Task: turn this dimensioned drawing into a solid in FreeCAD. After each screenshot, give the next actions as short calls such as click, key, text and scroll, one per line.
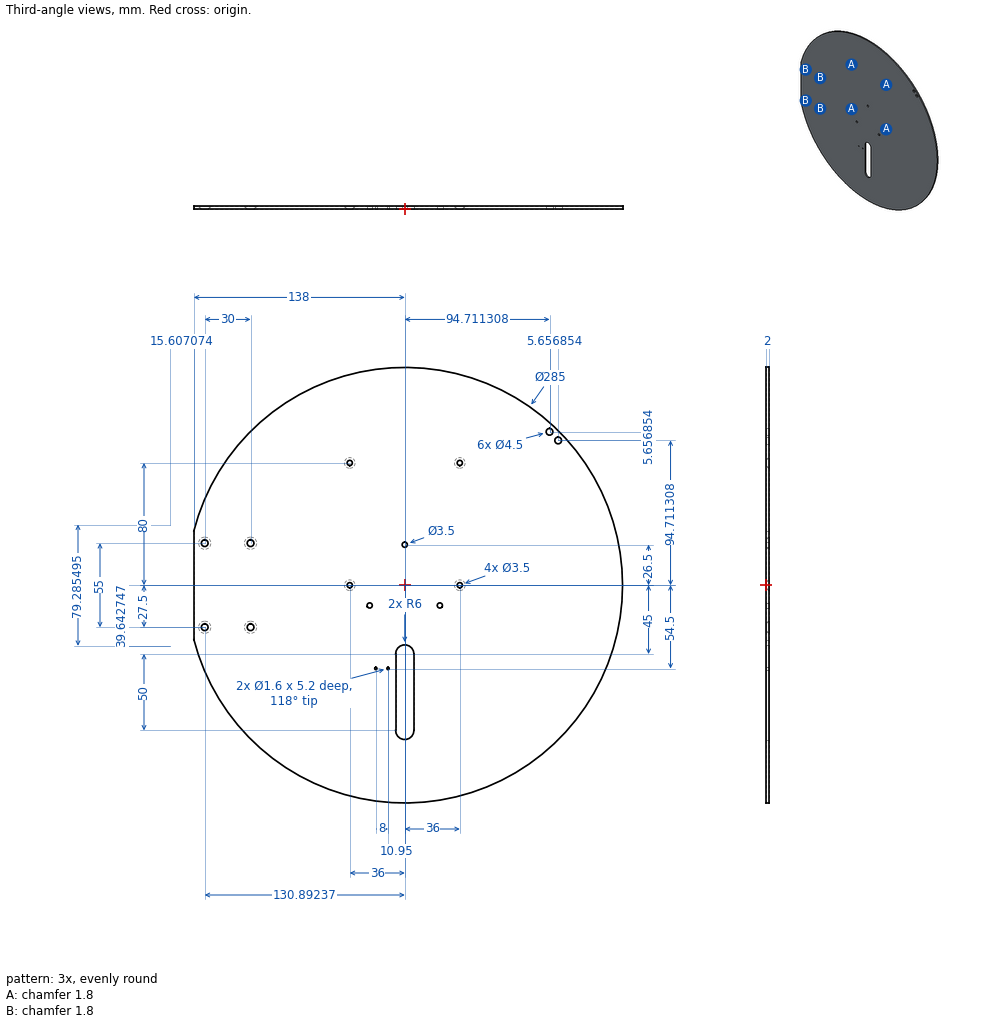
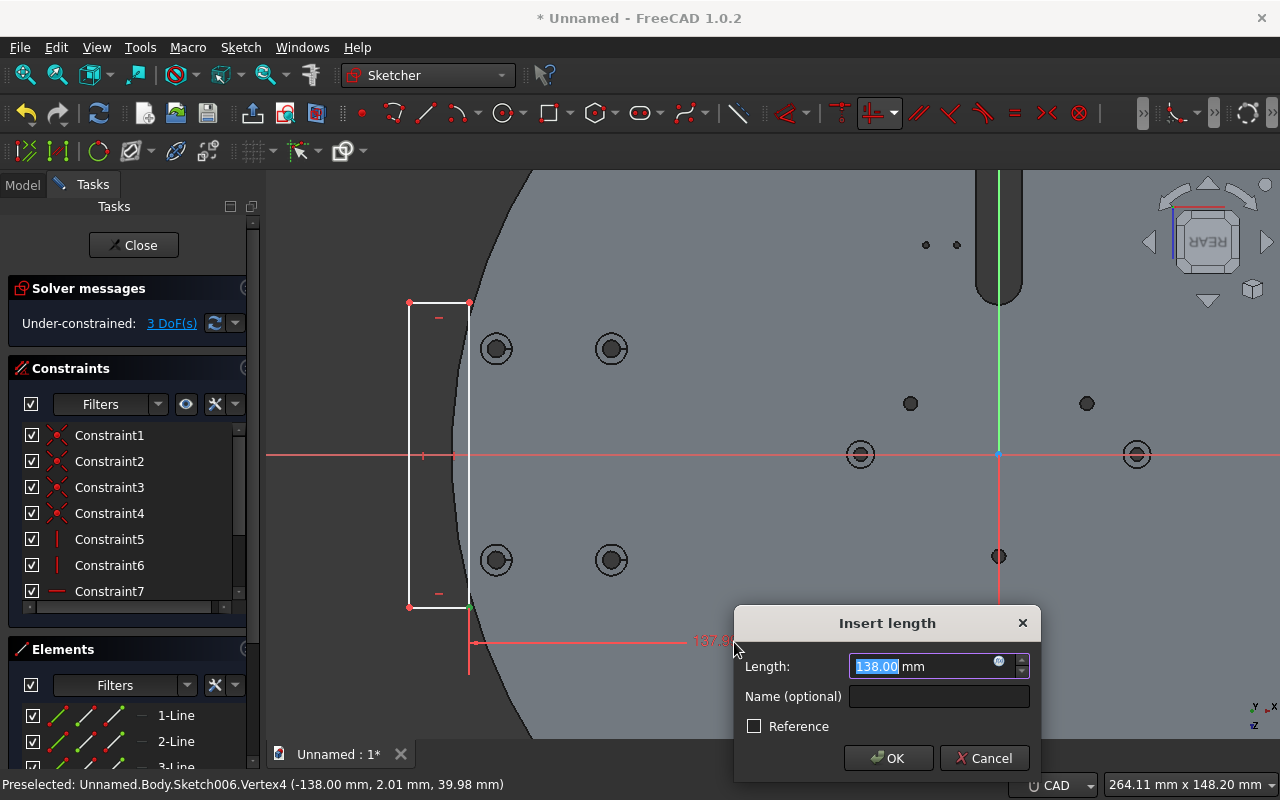
text(138)
key(Return)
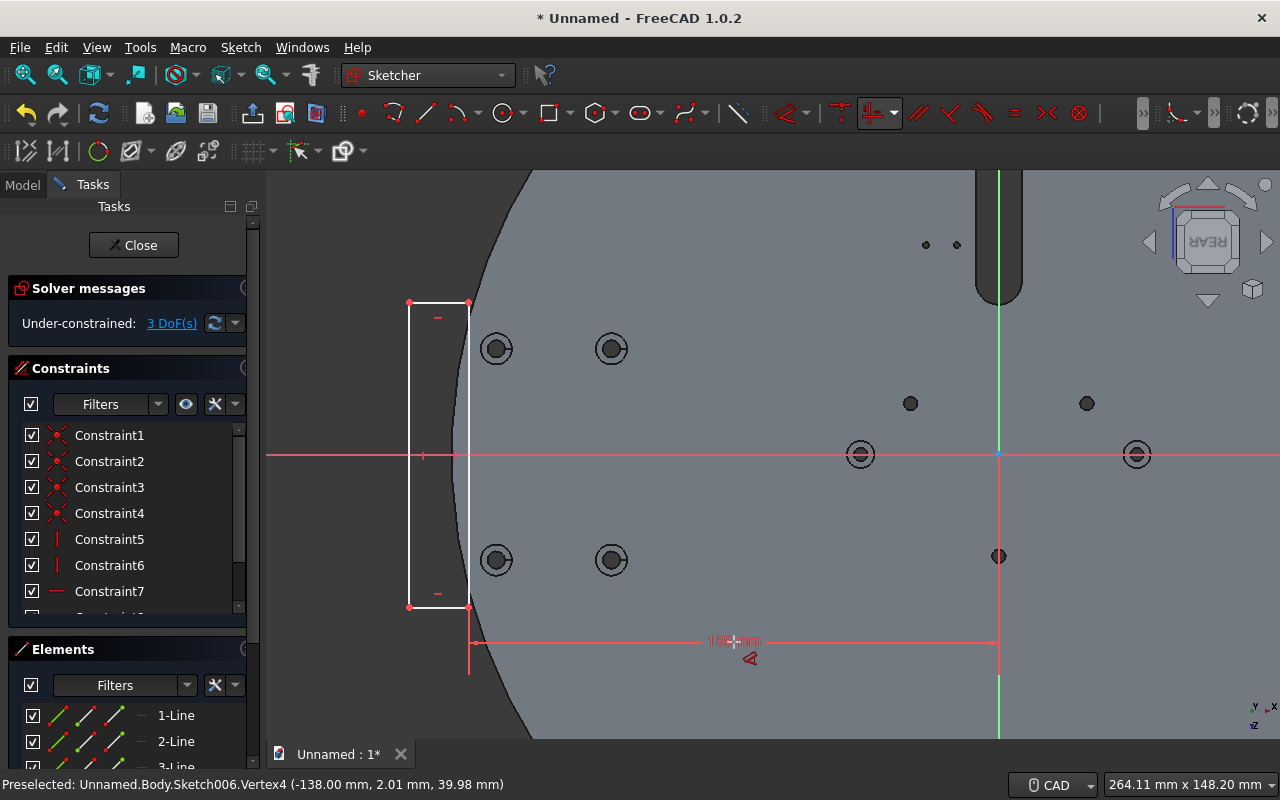
click(409, 395)
click(375, 385)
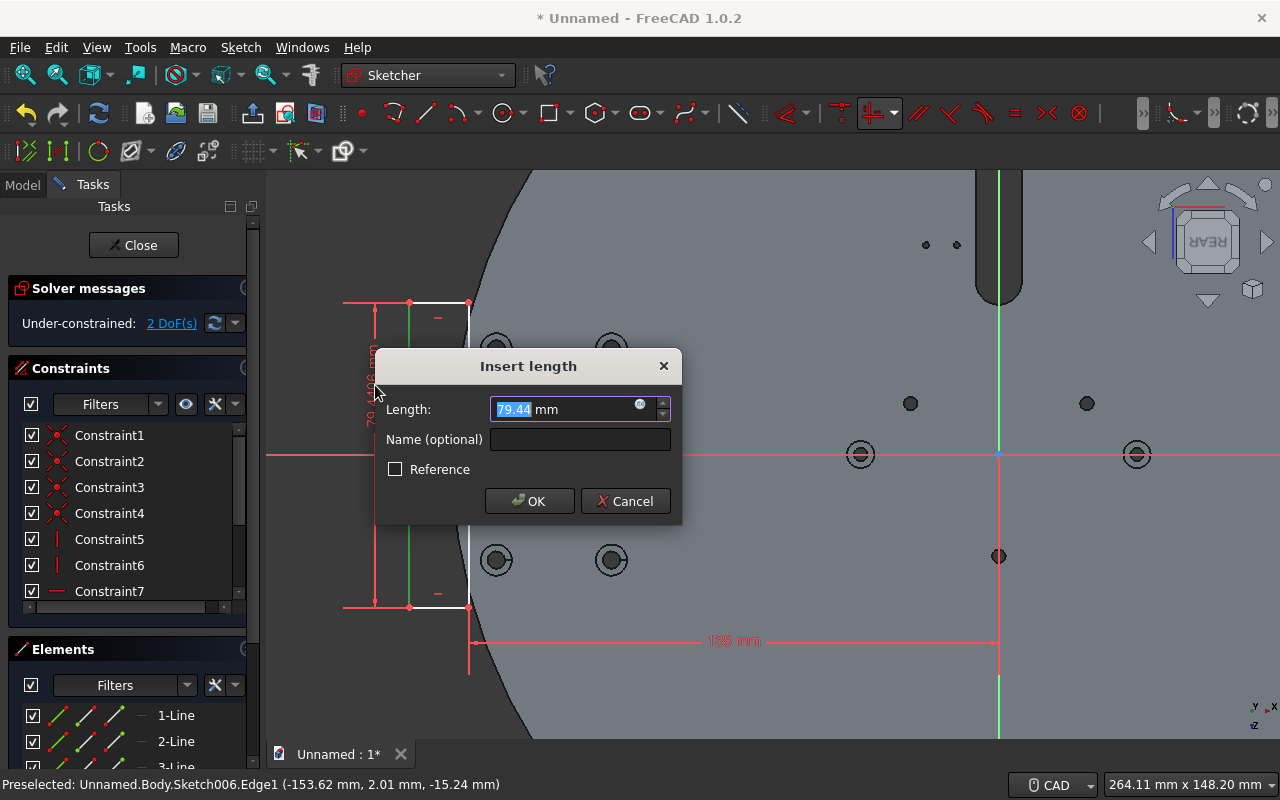
text(79.285495)
key(Return)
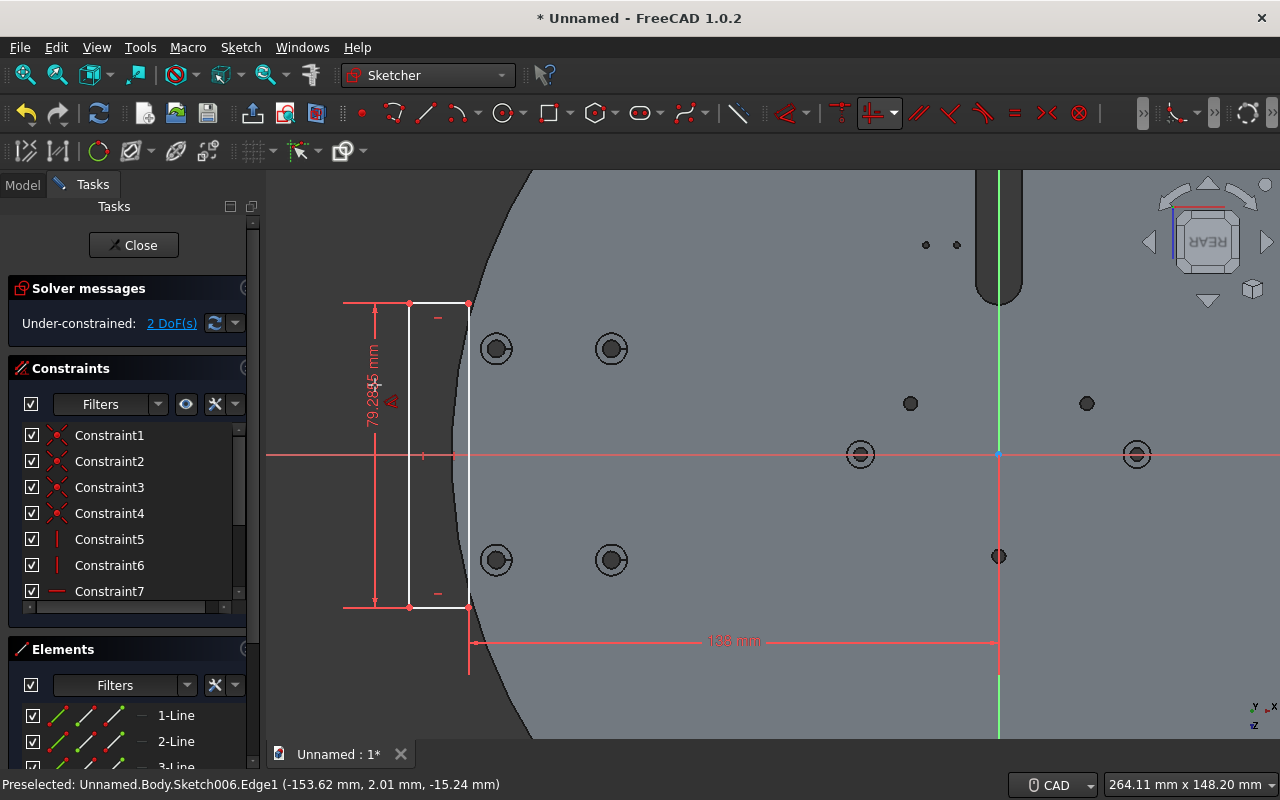
click(427, 608)
click(439, 642)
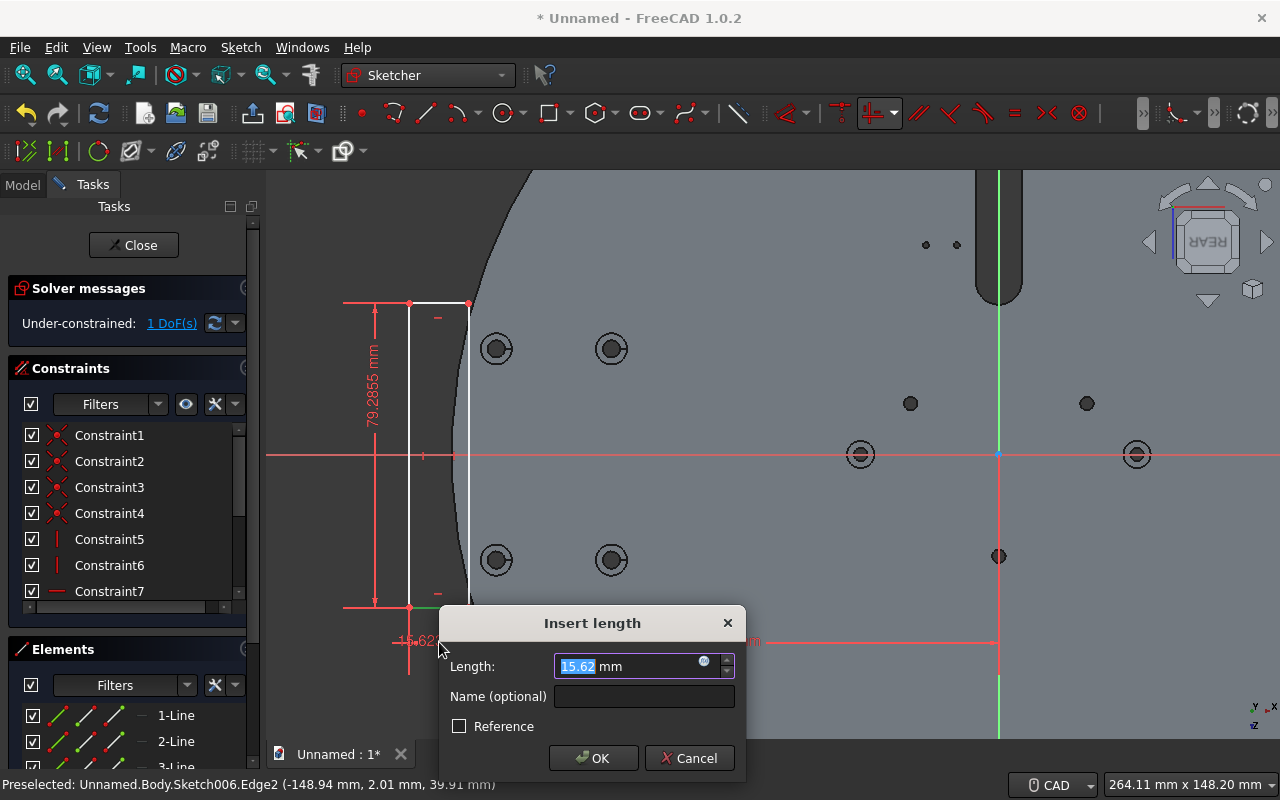
text(15.607074)
key(Return)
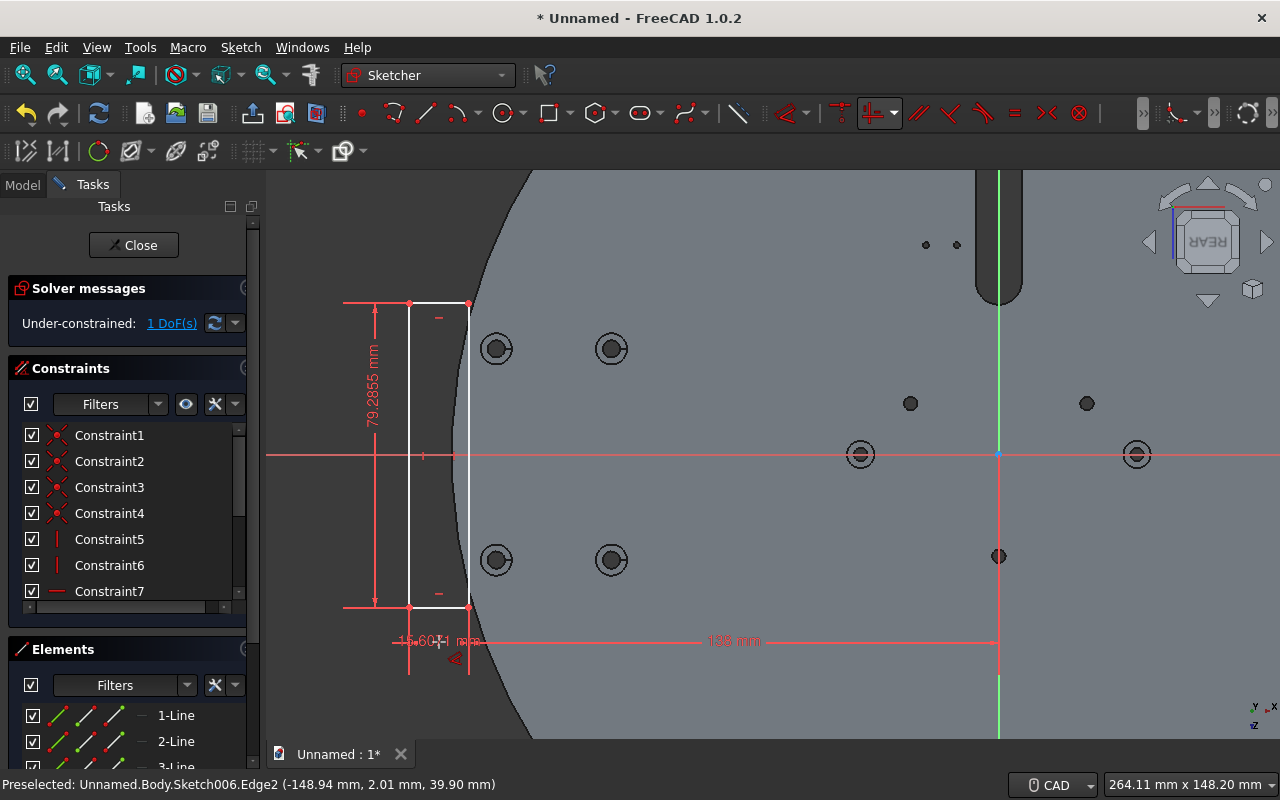
click(409, 303)
click(375, 344)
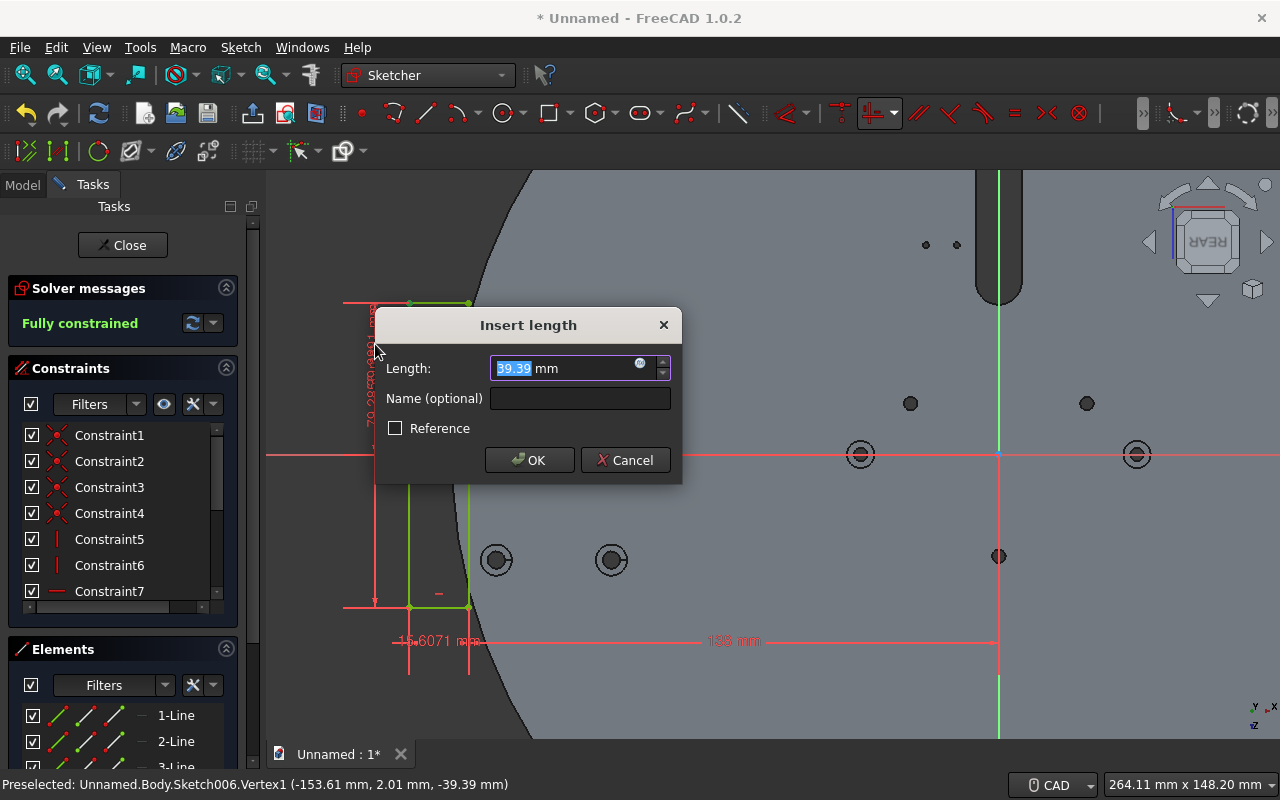
text(39.642747)
key(Return)
key(Escape)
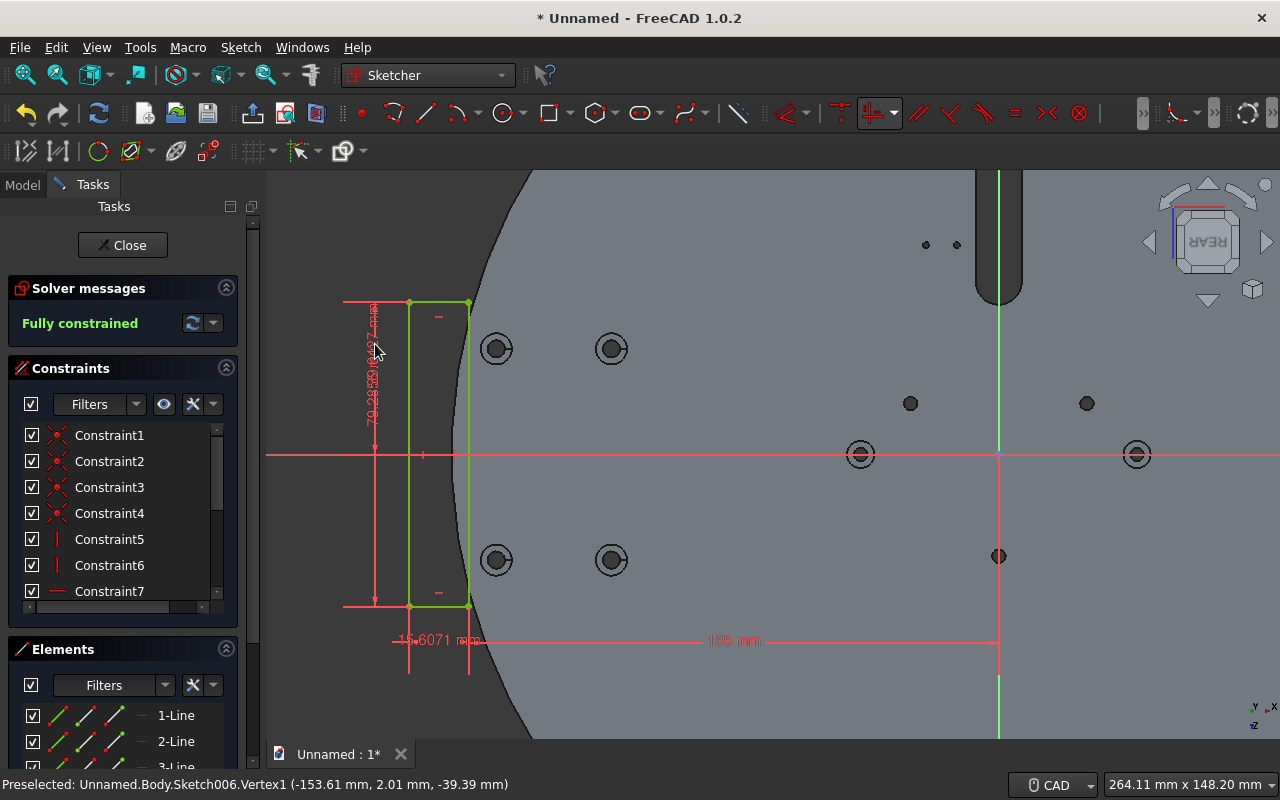
click(123, 245)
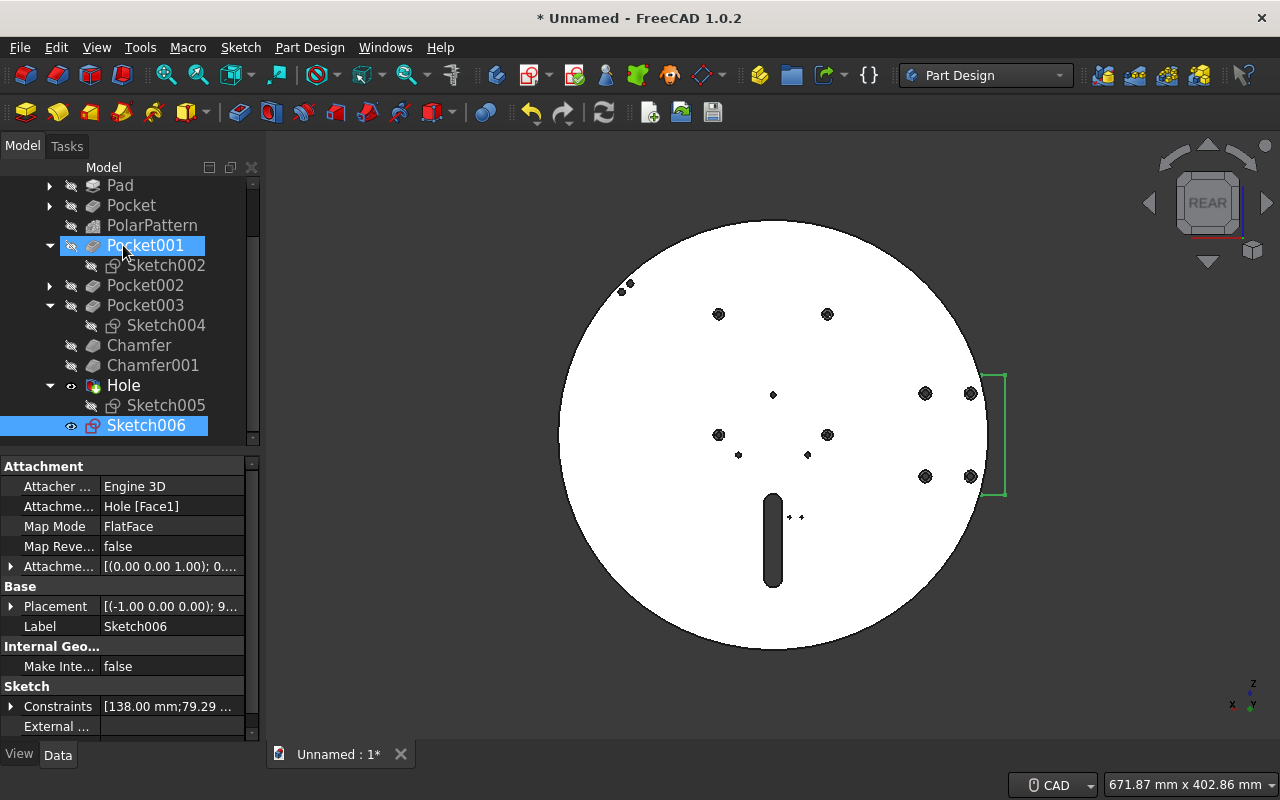
click(240, 112)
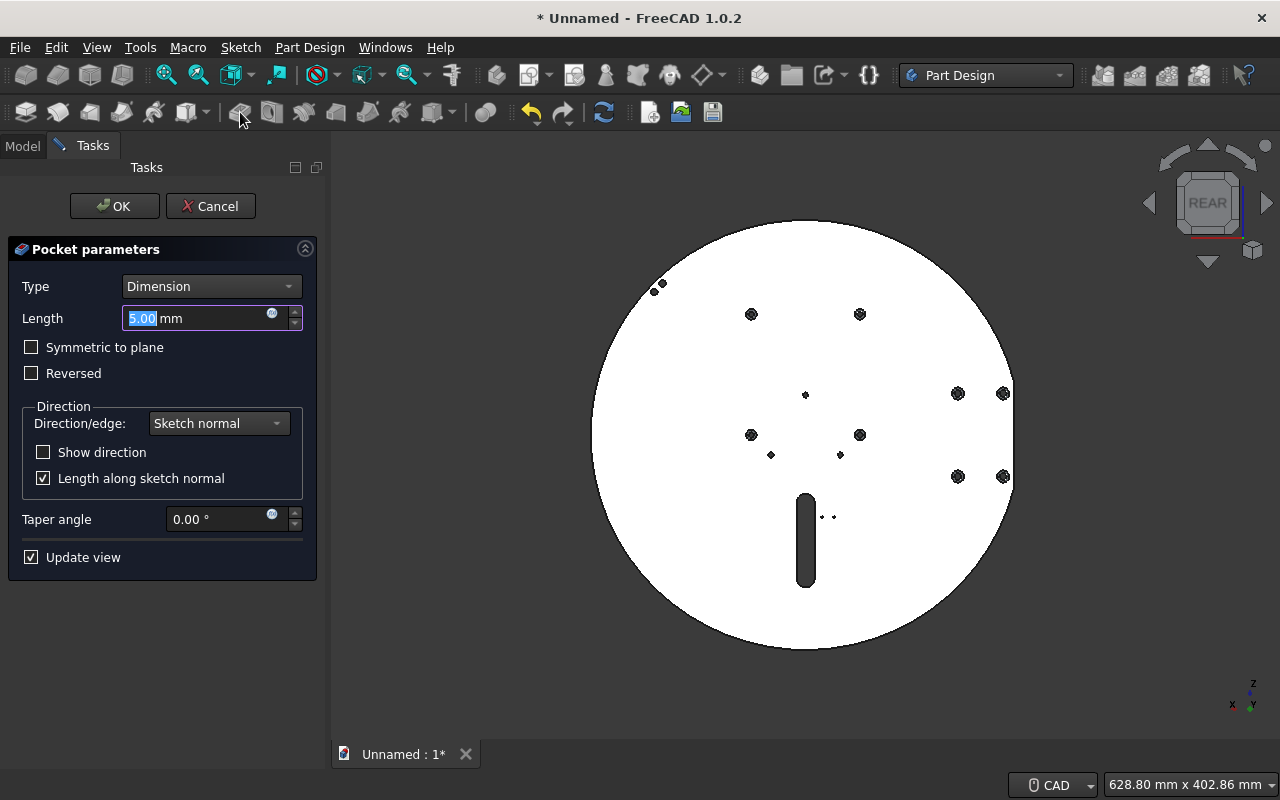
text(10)
key(Tab)